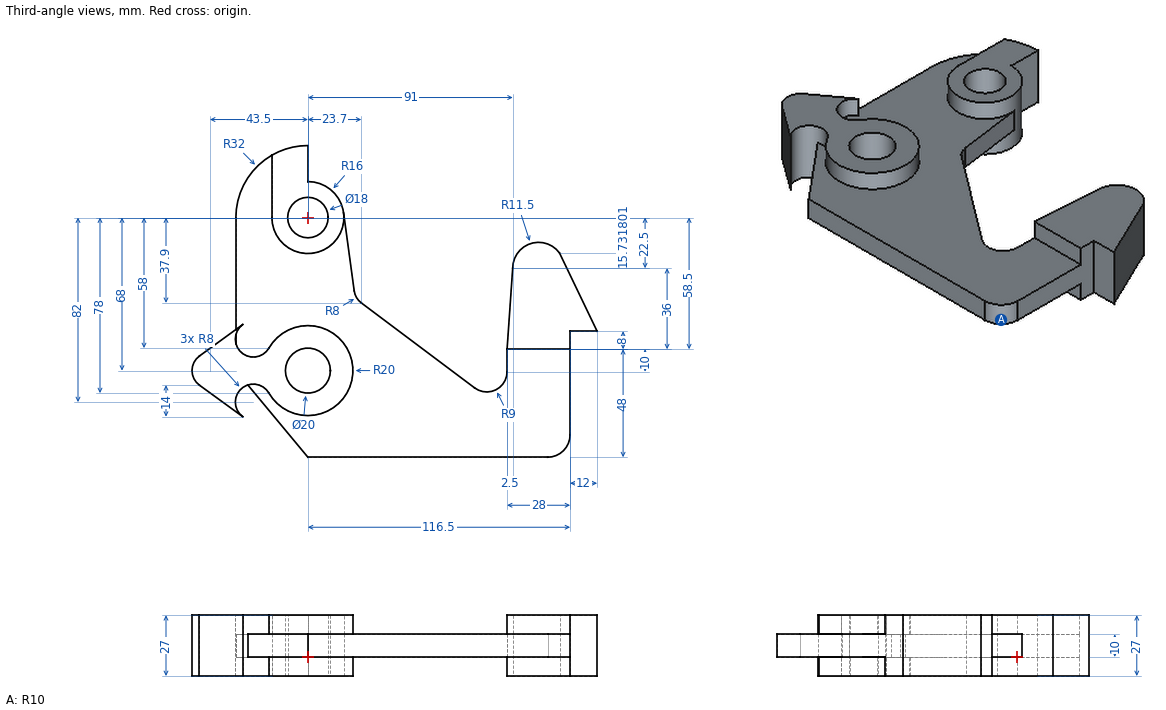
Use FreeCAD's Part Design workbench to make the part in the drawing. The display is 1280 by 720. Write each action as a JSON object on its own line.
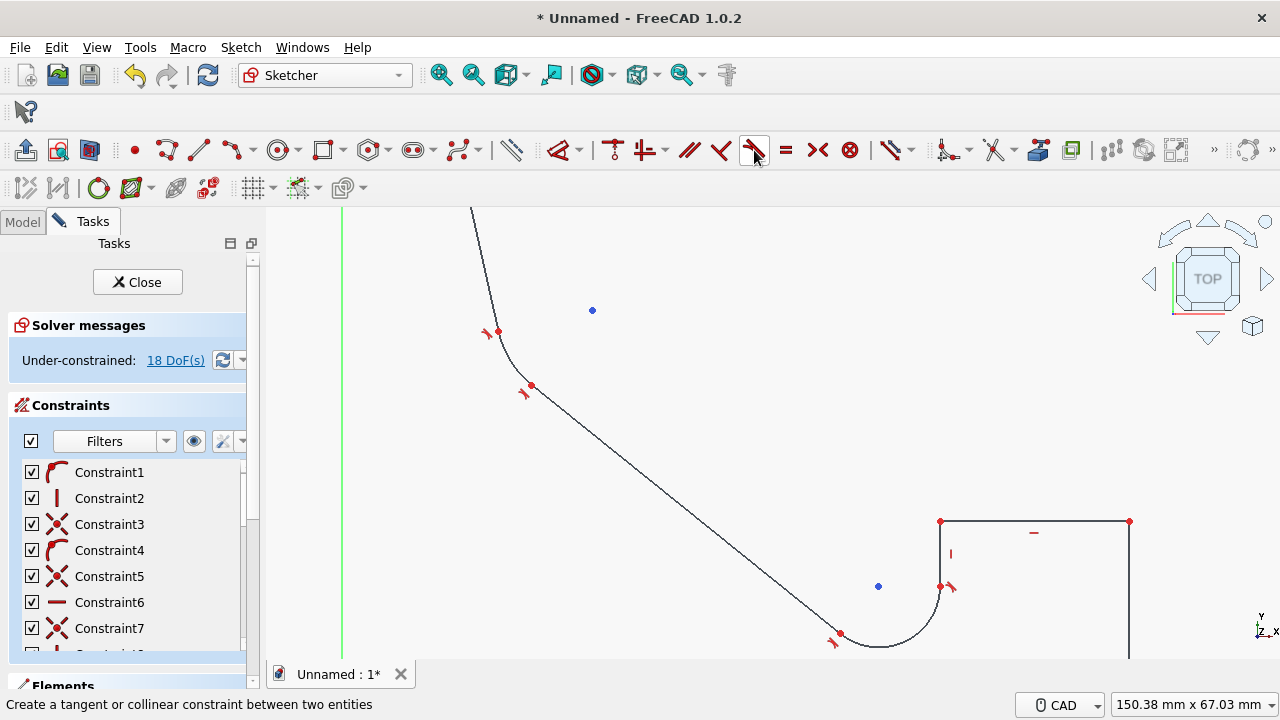
{"action": "left_click", "coordinate": [484, 265]}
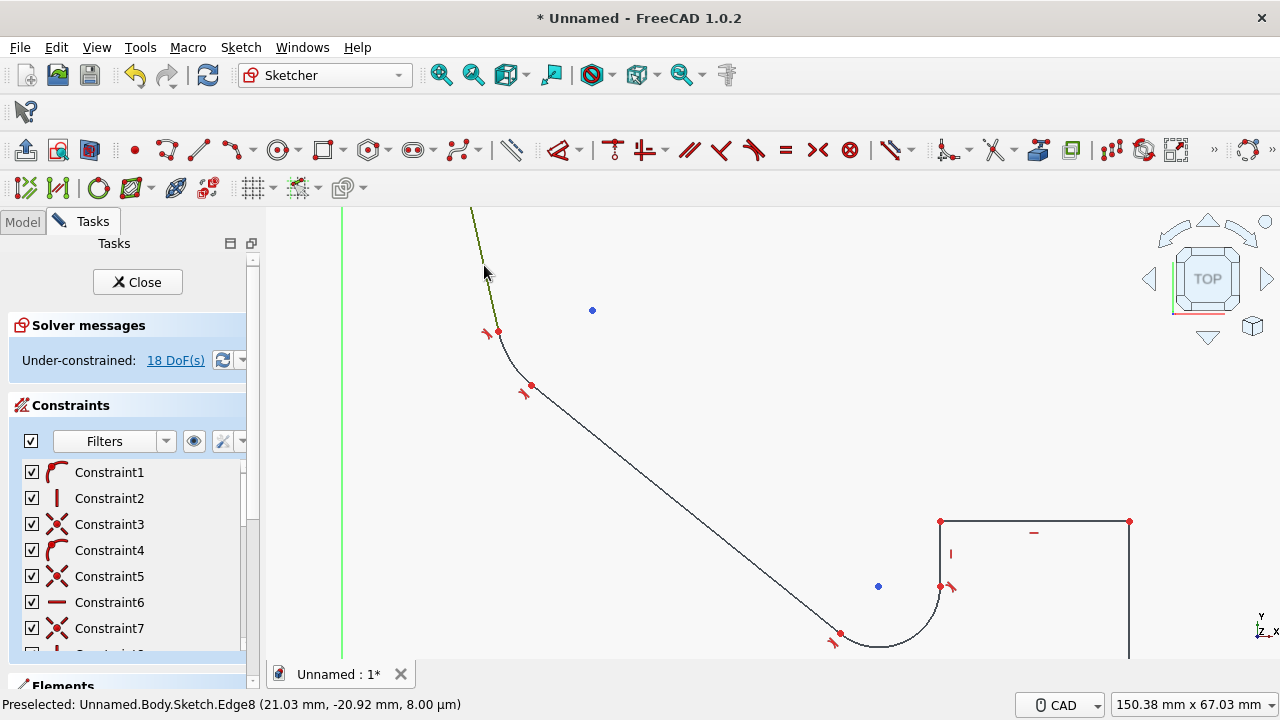
{"action": "scroll", "coordinate": [738, 458], "scroll_direction": "down", "scroll_amount": 6}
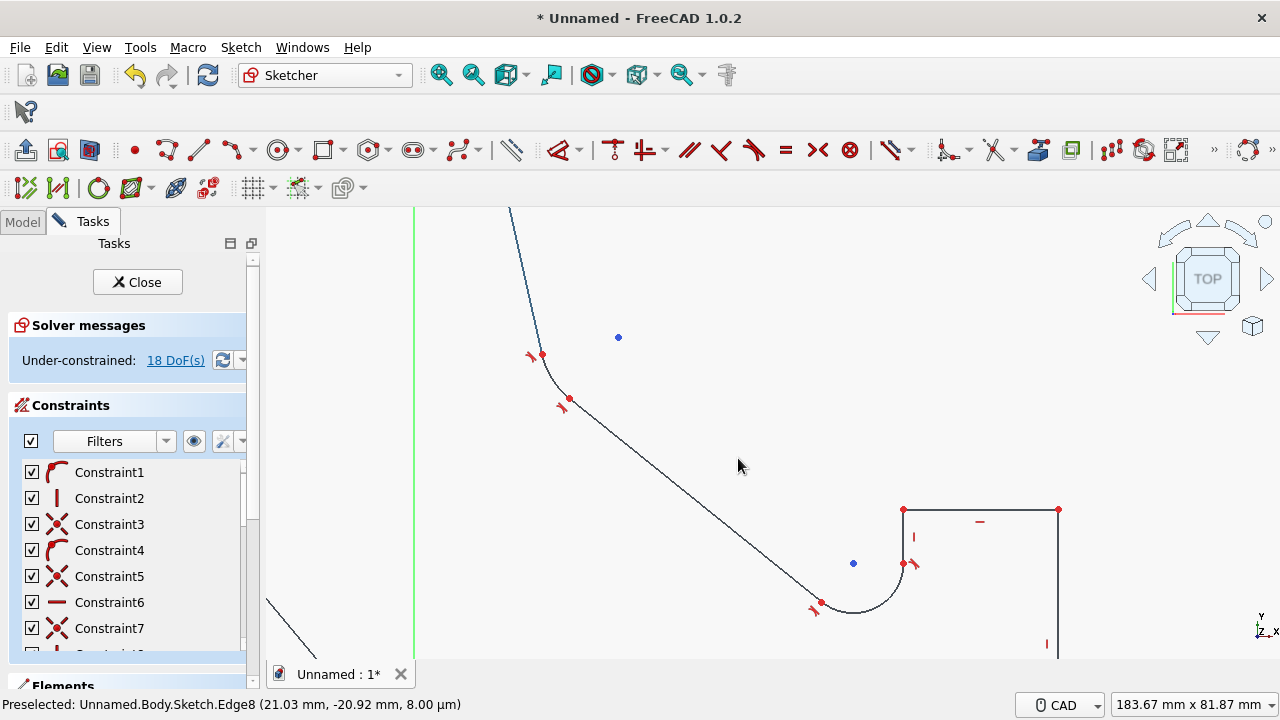
{"action": "left_click", "coordinate": [647, 341]}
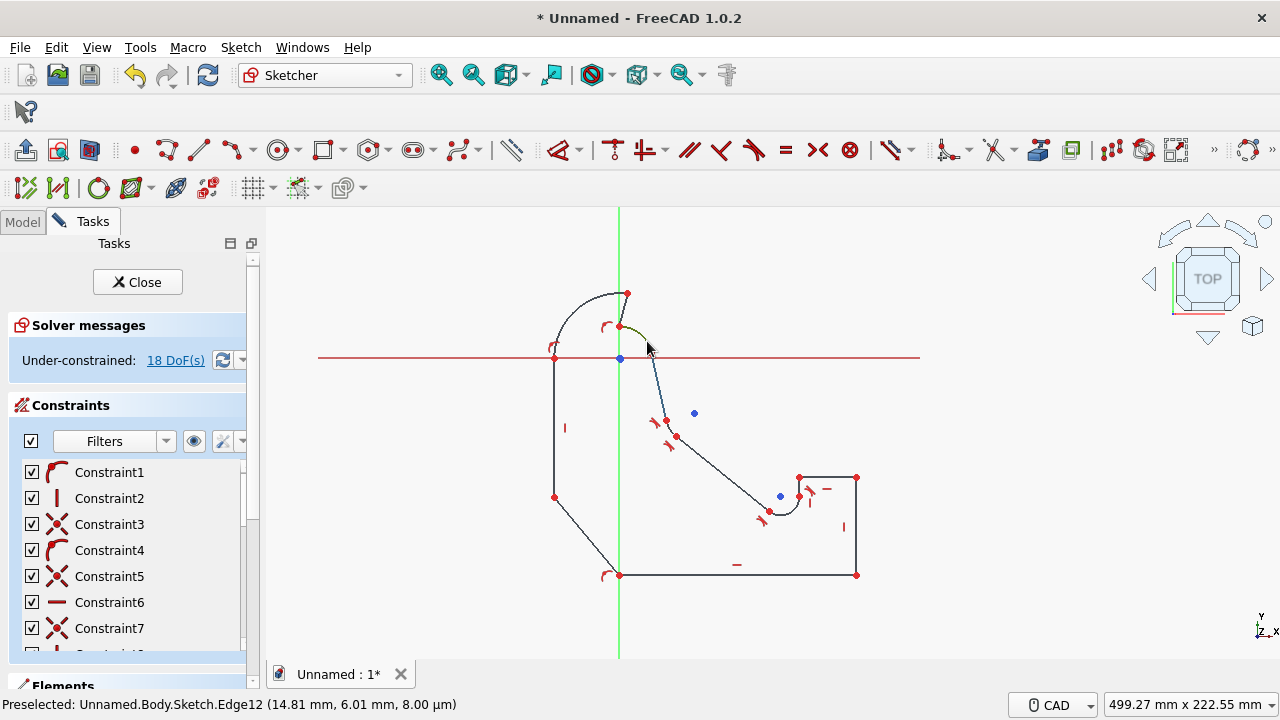
{"action": "left_click", "coordinate": [754, 150]}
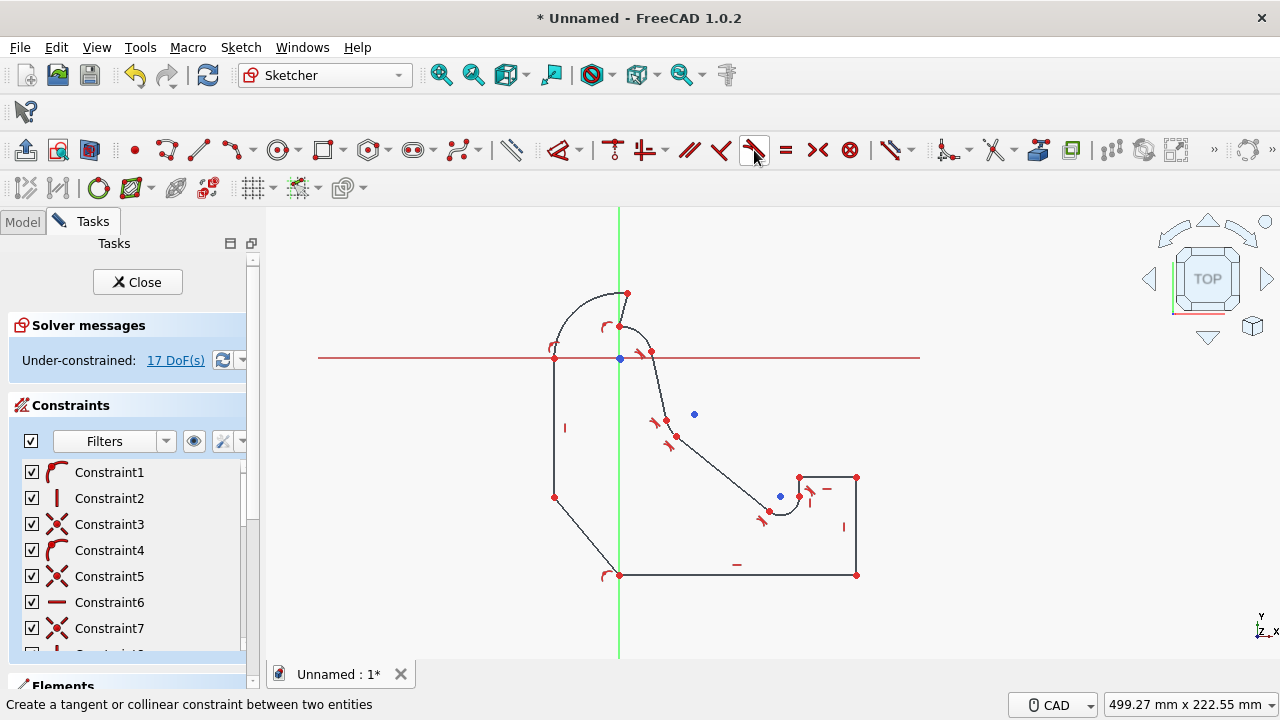
{"action": "scroll", "coordinate": [622, 317], "scroll_direction": "up", "scroll_amount": 2}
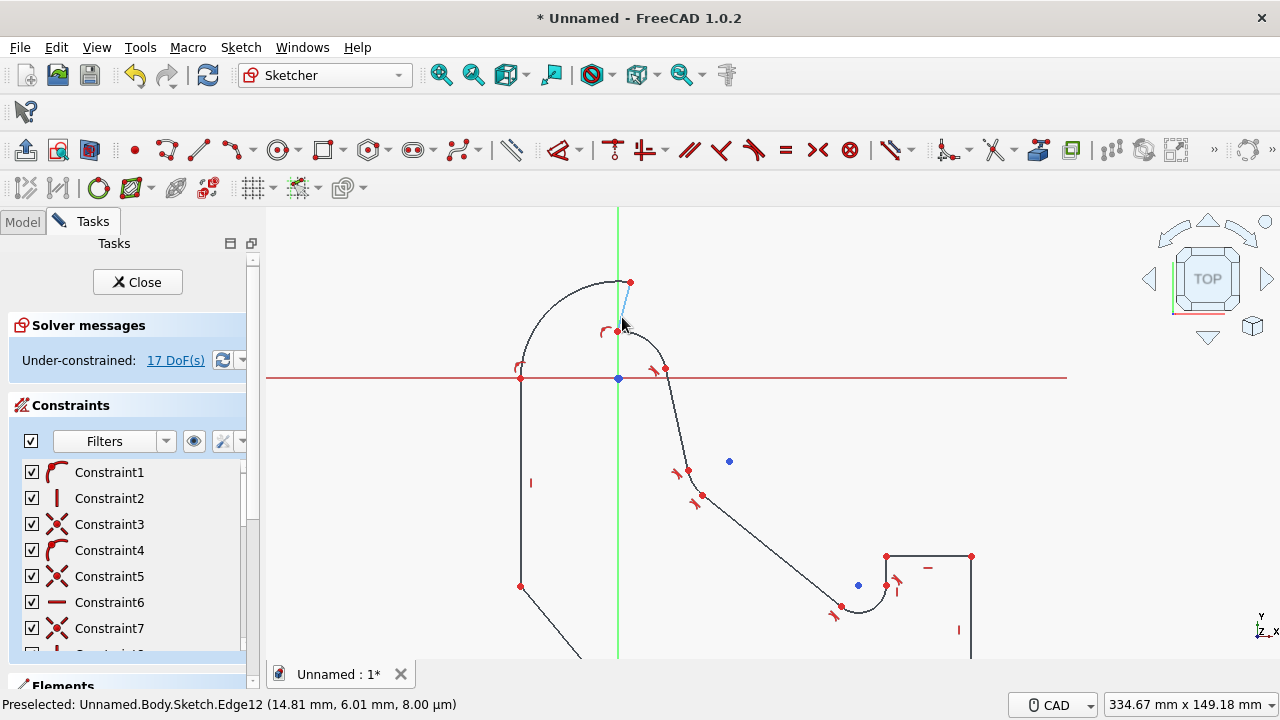
{"action": "left_click", "coordinate": [621, 317]}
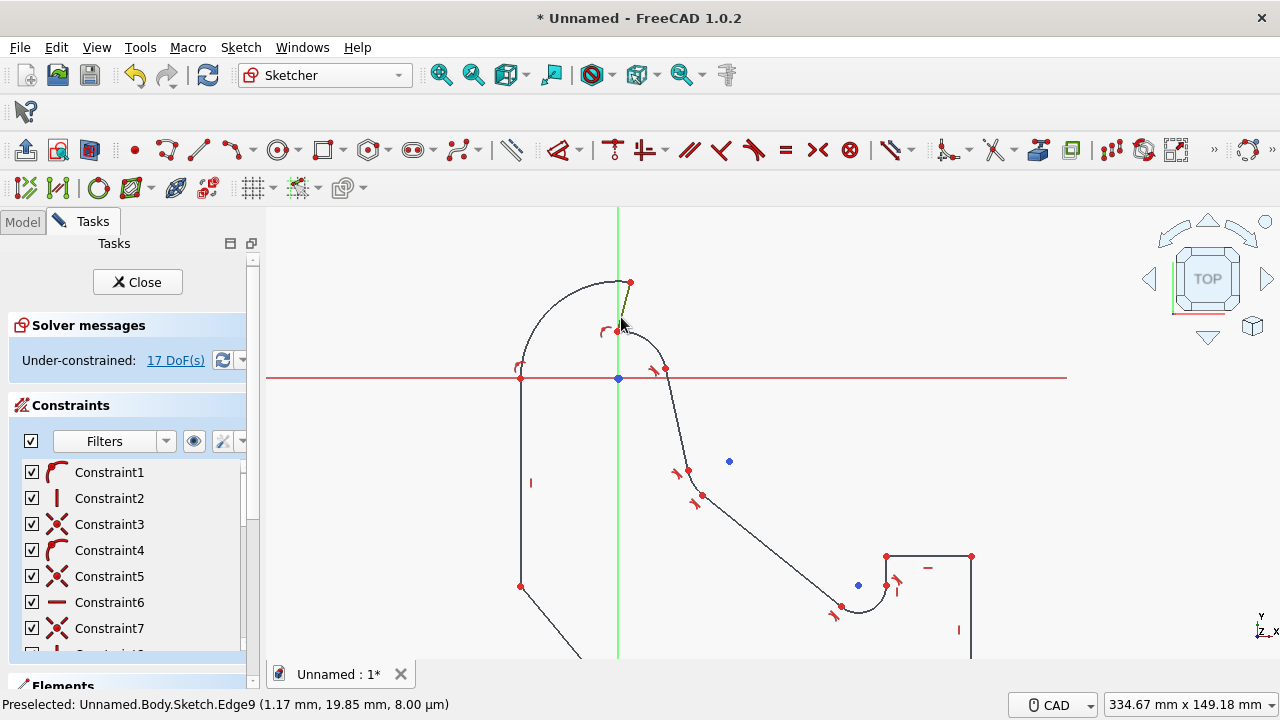
{"action": "key", "text": "v"}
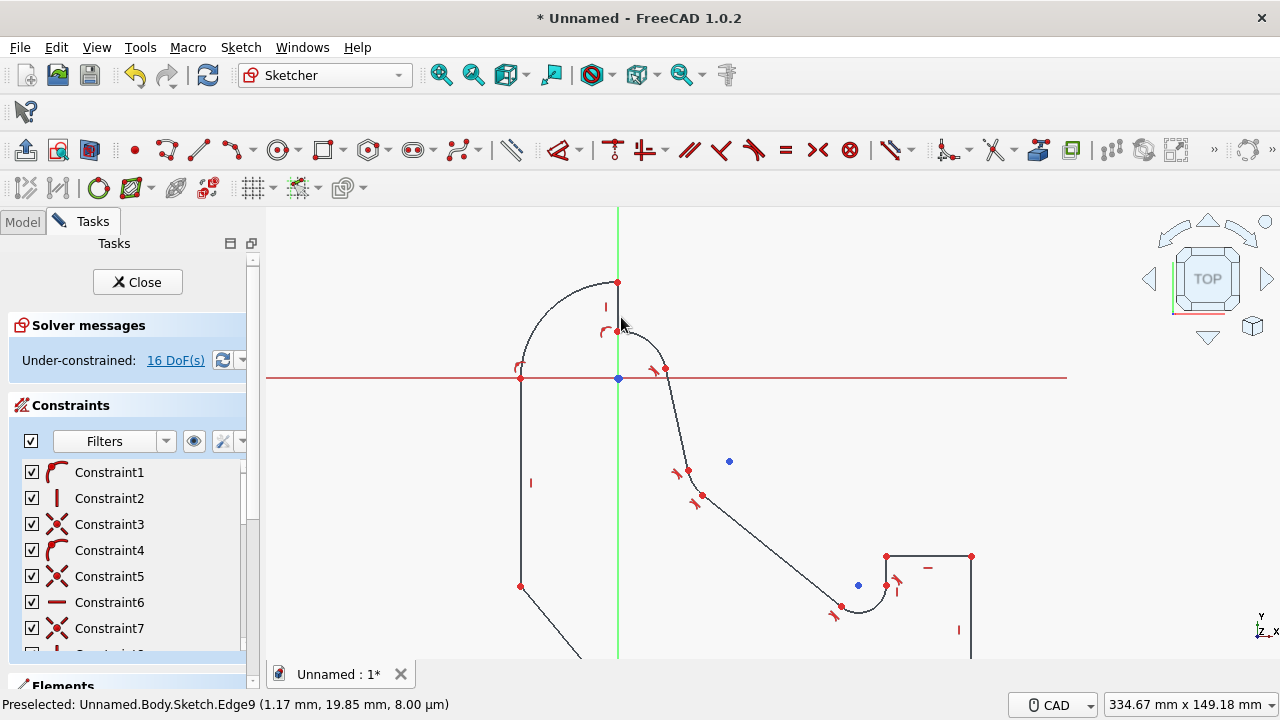
{"action": "left_click", "coordinate": [658, 350]}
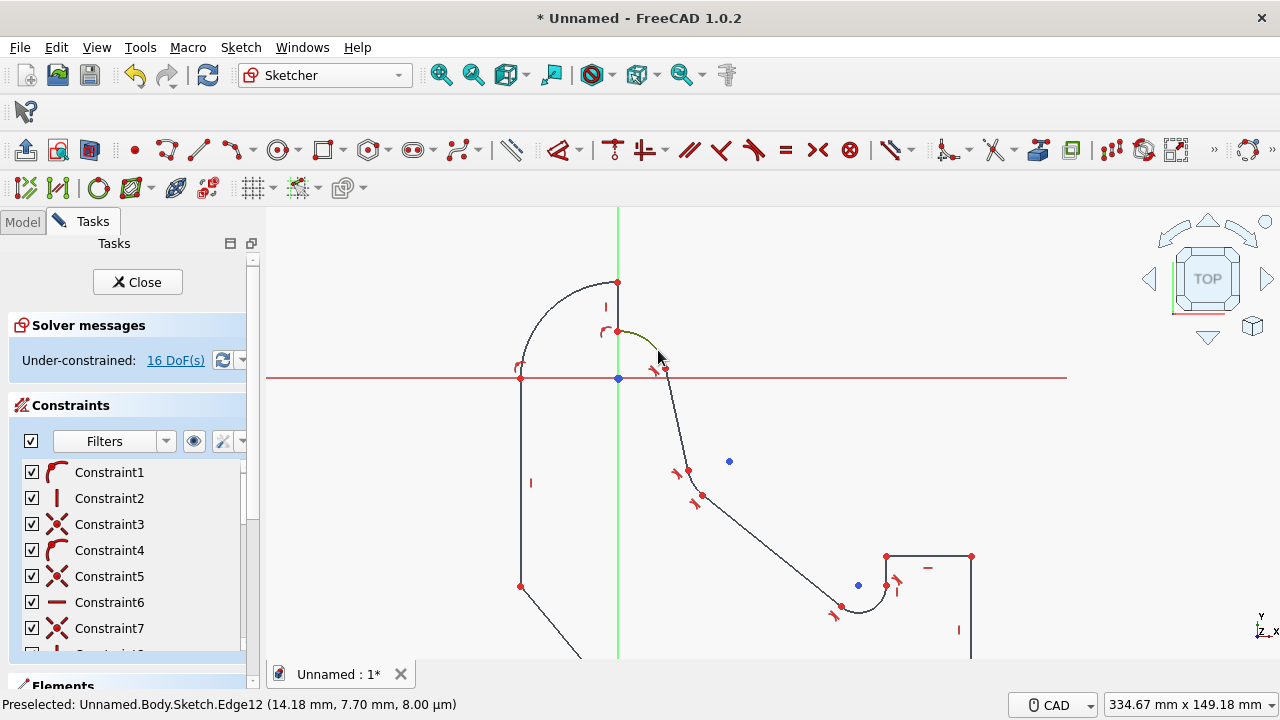
{"action": "left_click", "coordinate": [574, 293]}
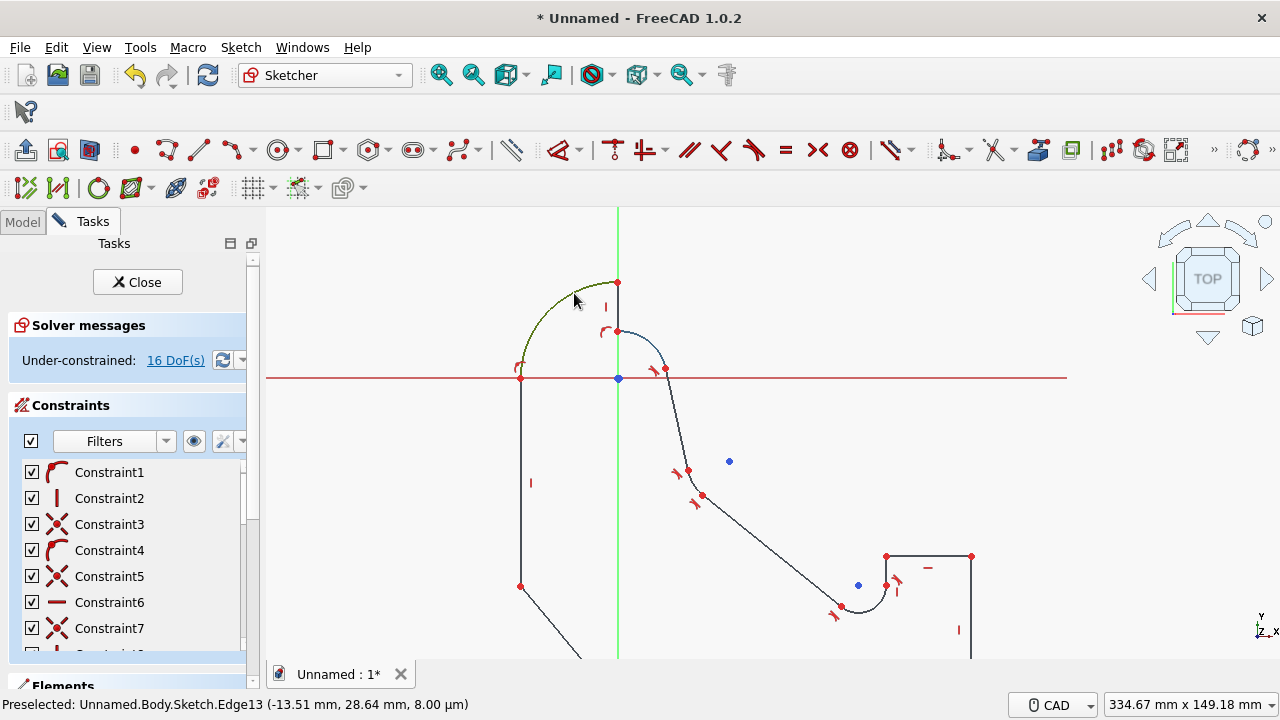
{"action": "left_click", "coordinate": [614, 150]}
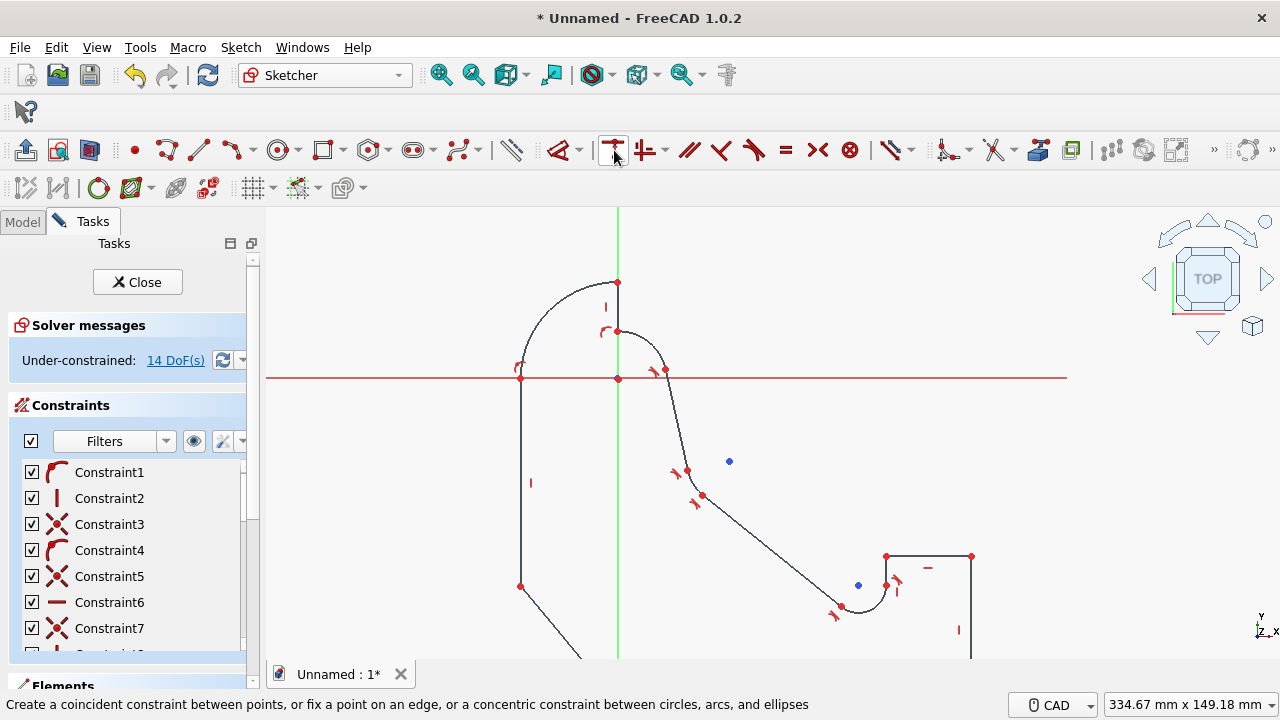
{"action": "scroll", "coordinate": [618, 379], "scroll_direction": "up", "scroll_amount": 2}